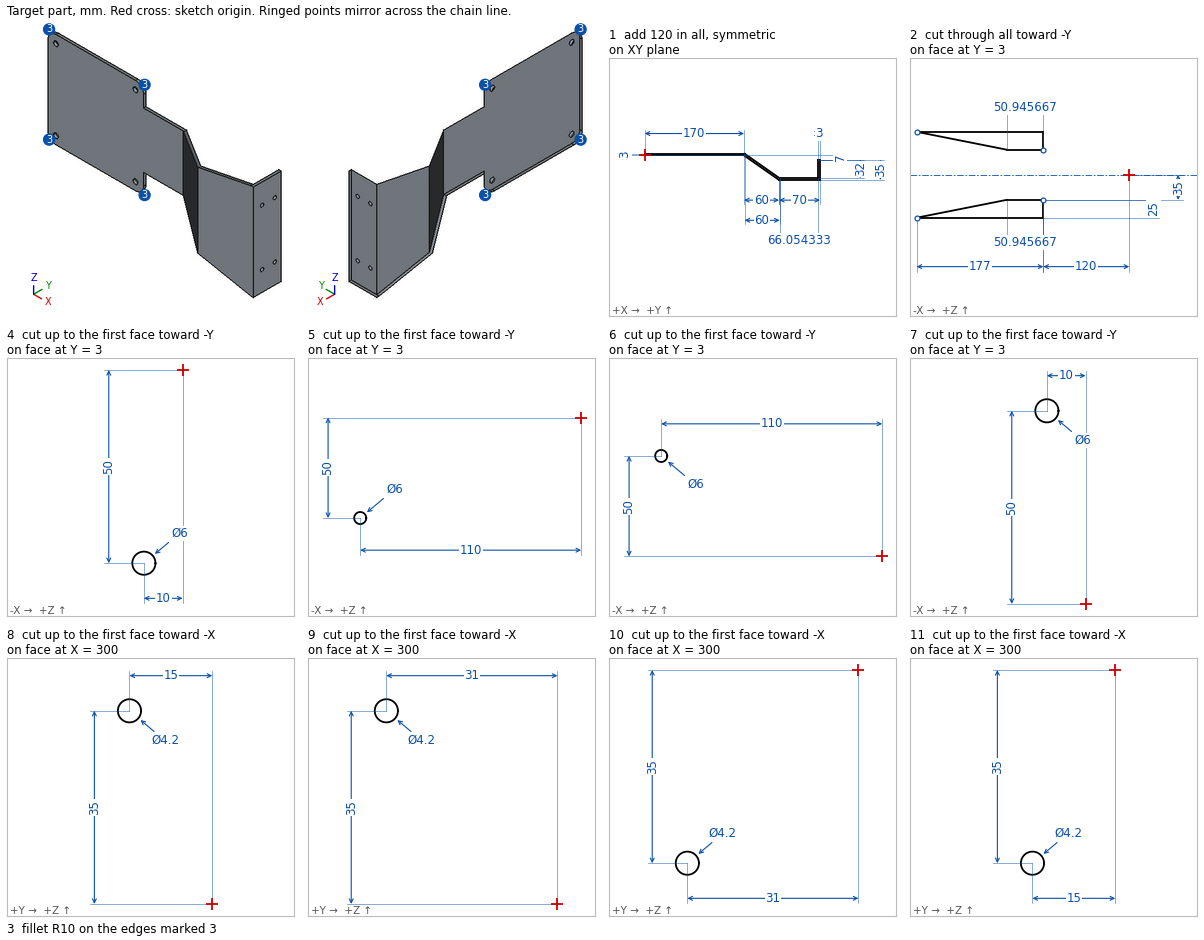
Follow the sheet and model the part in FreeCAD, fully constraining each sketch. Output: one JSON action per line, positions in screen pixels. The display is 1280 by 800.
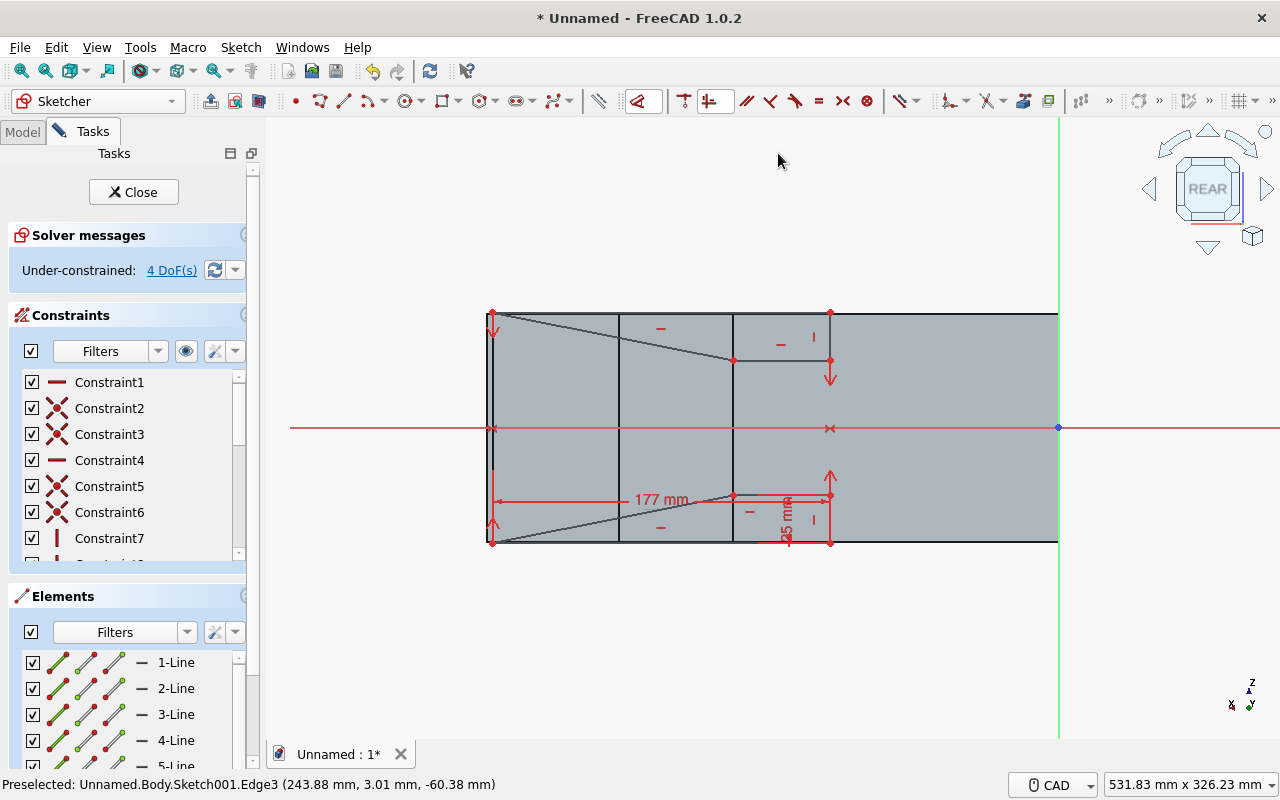
{"action": "left_click", "coordinate": [830, 495]}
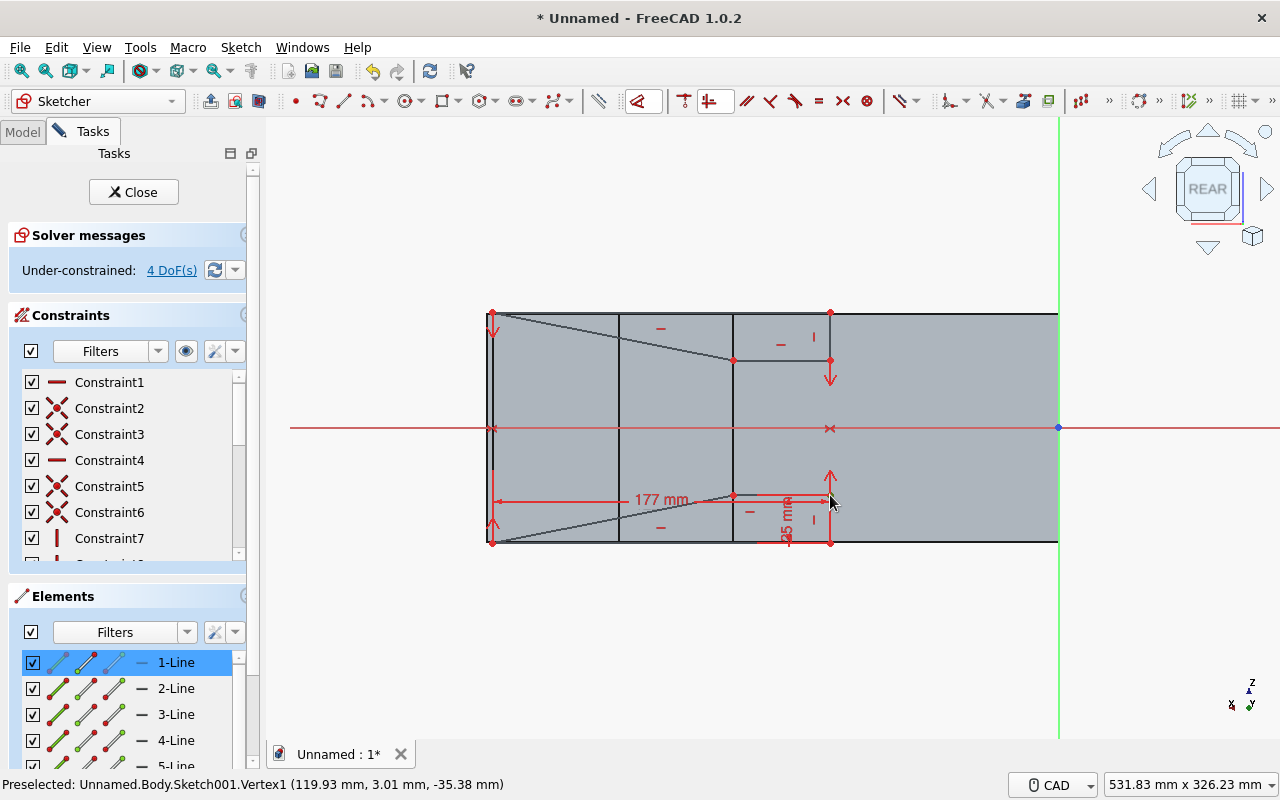
{"action": "key", "text": "i"}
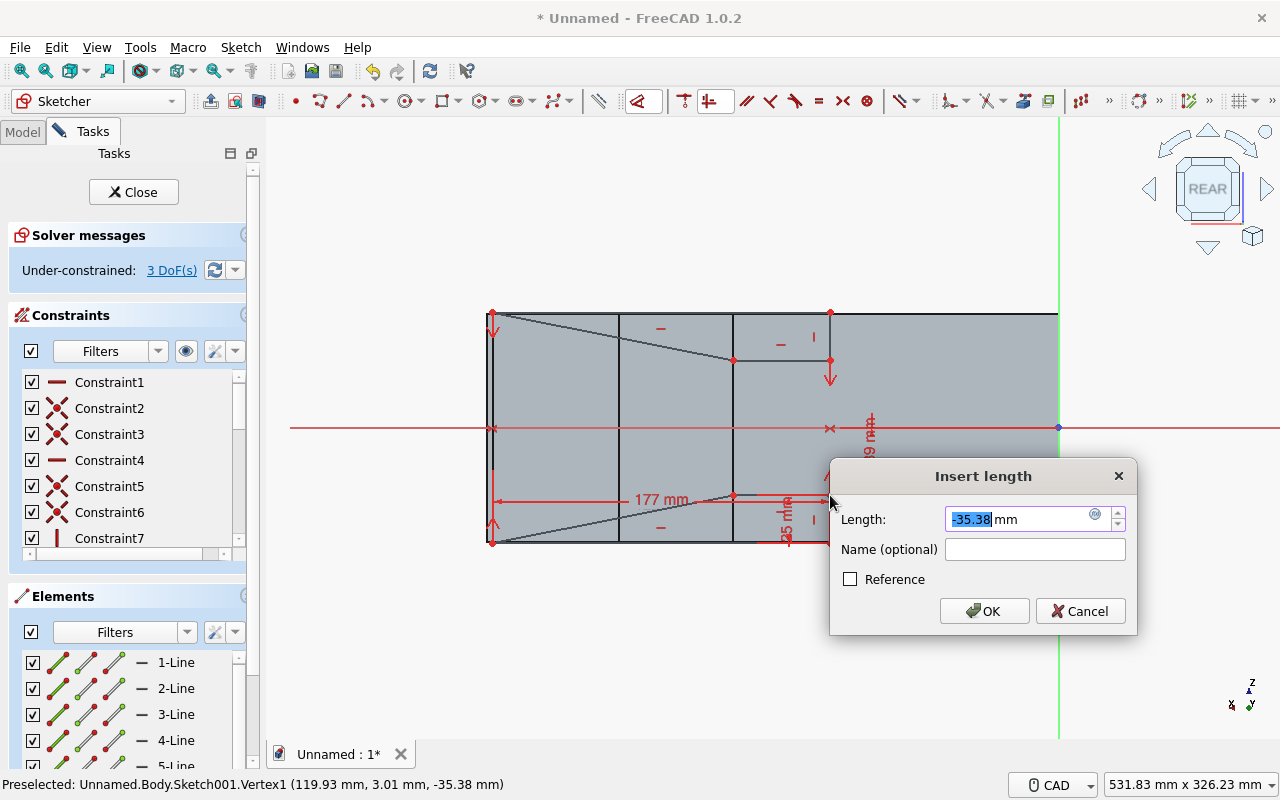
{"action": "type", "text": "-35"}
{"action": "key", "text": "Return"}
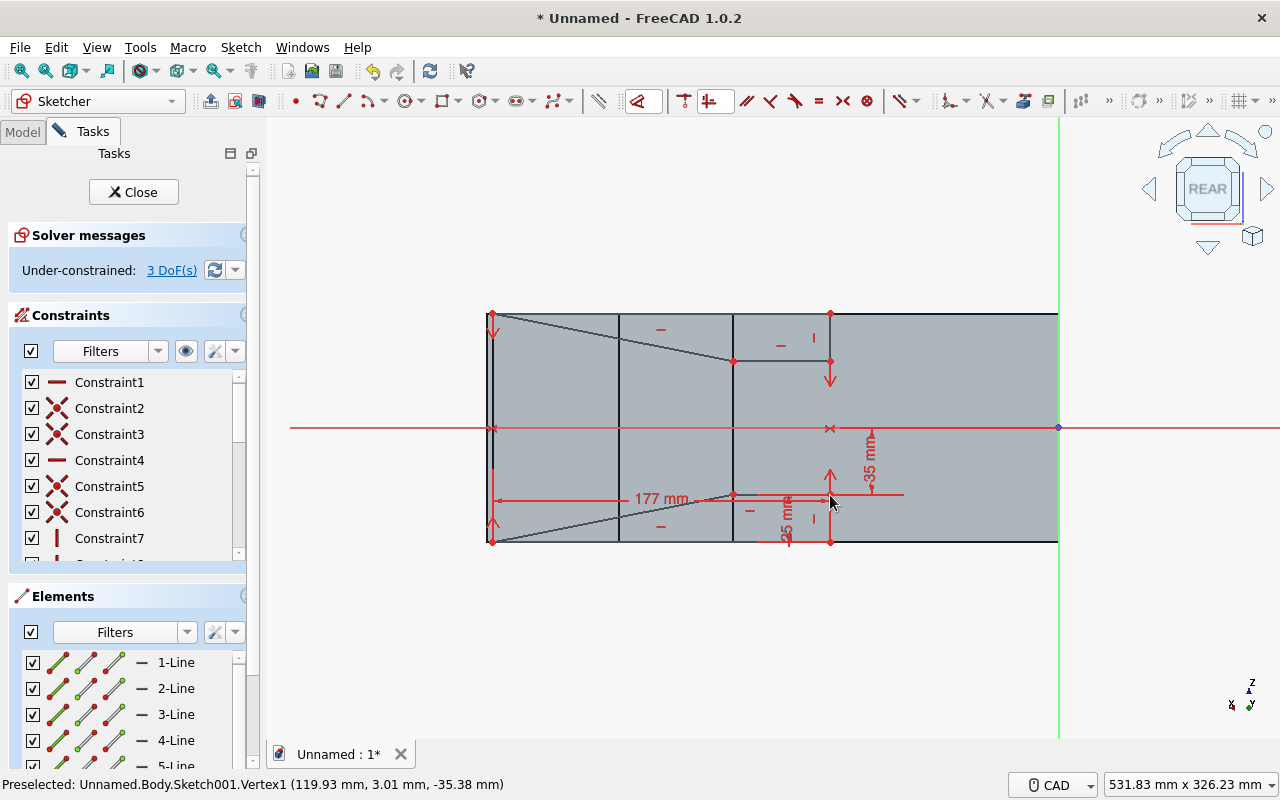
{"action": "left_click", "coordinate": [830, 495]}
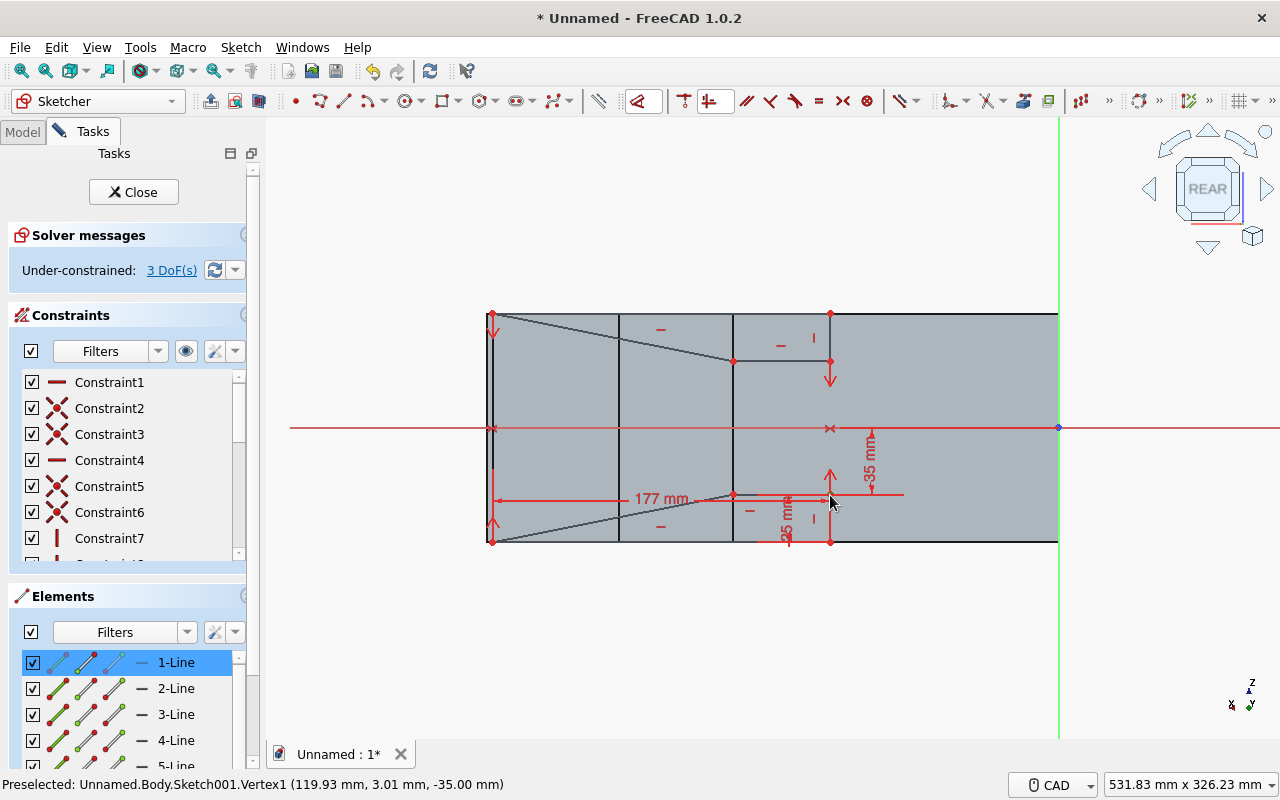
{"action": "left_click", "coordinate": [656, 102]}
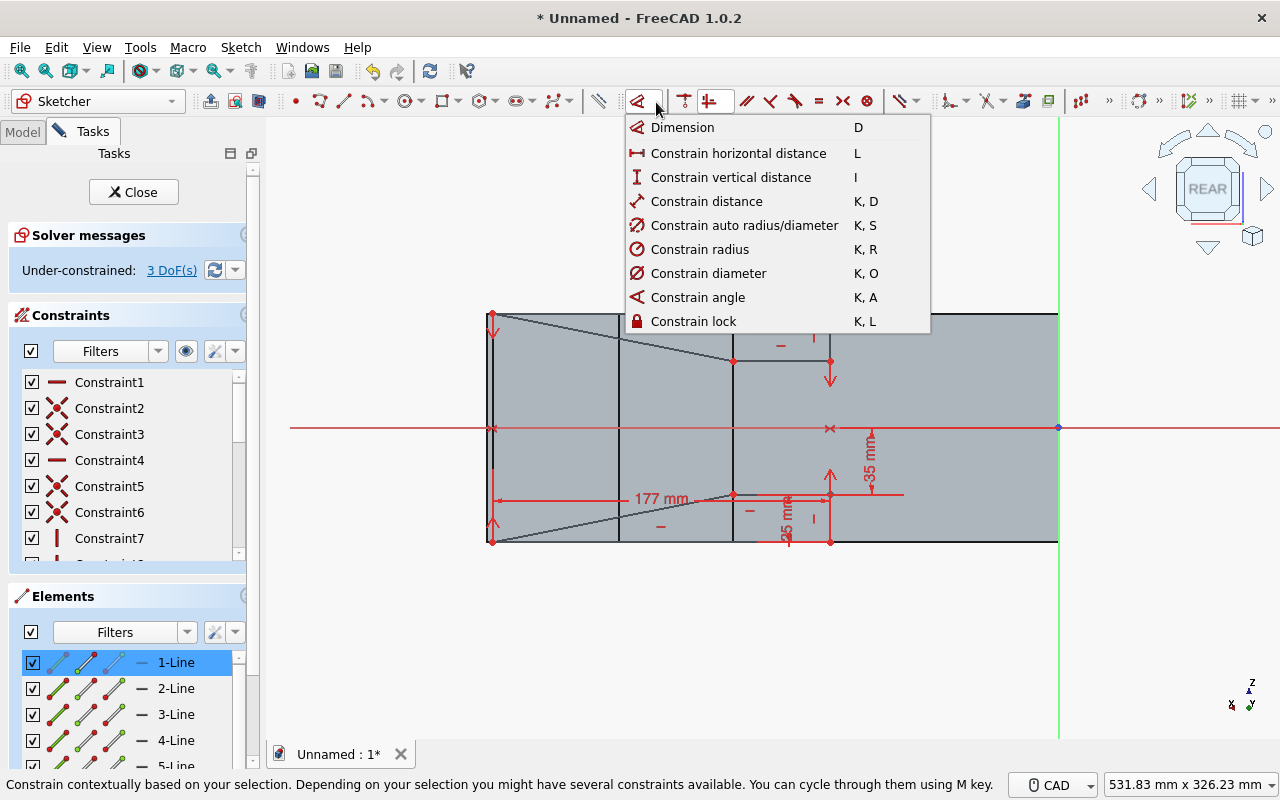
{"action": "left_click", "coordinate": [778, 153]}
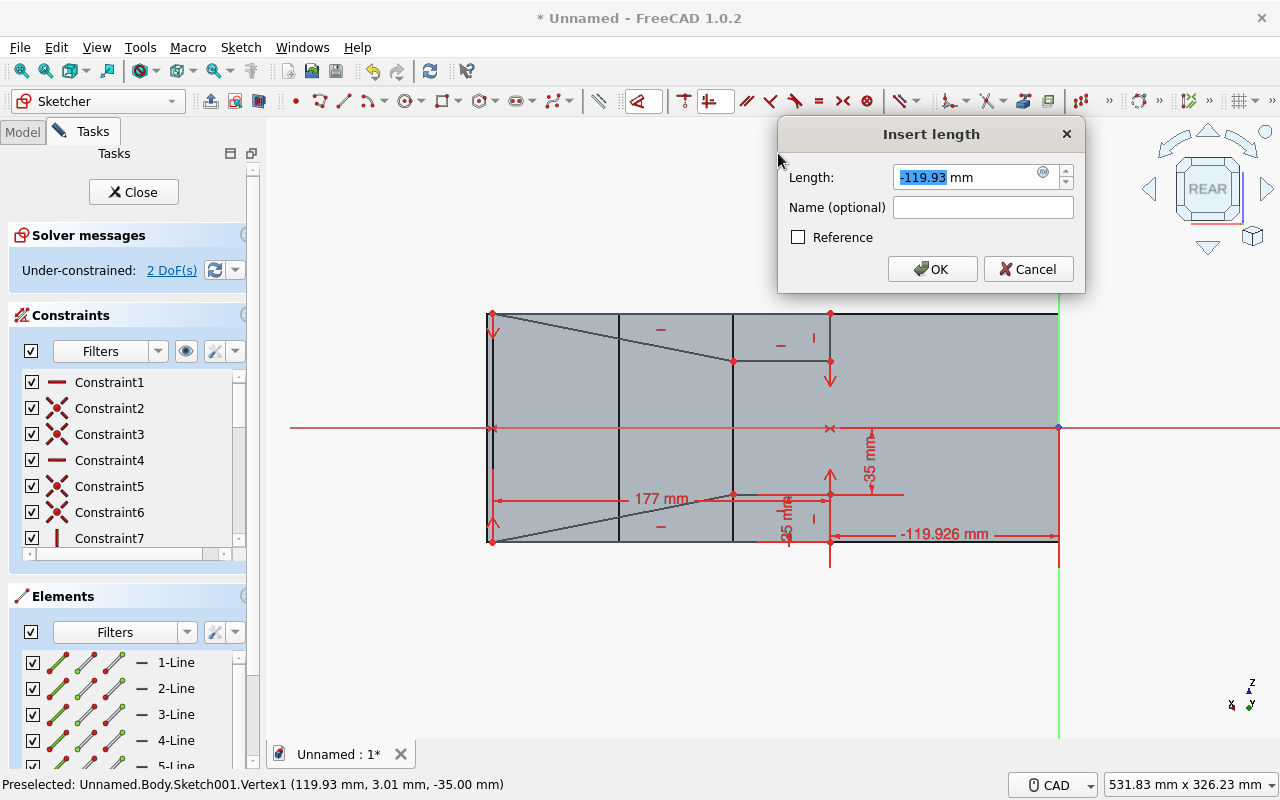
{"action": "type", "text": "-120"}
{"action": "key", "text": "Return"}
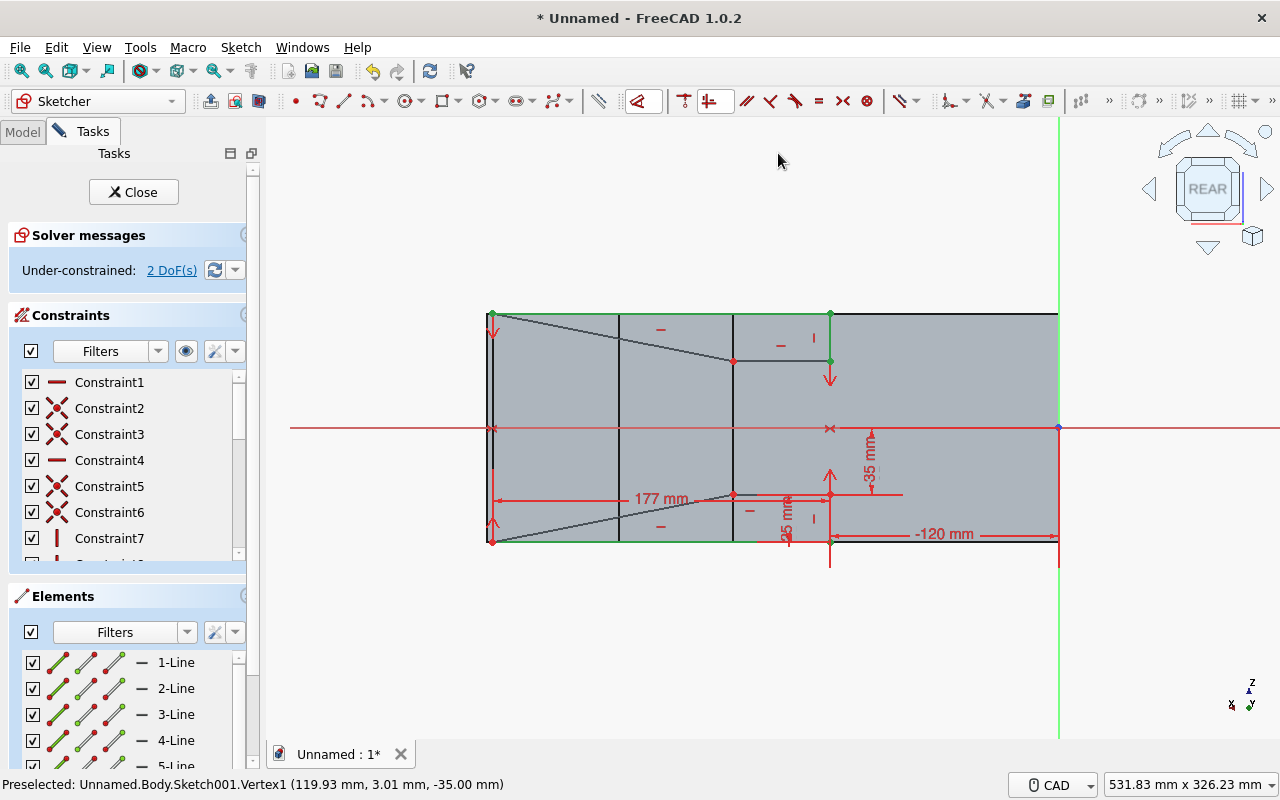
{"action": "left_click", "coordinate": [801, 495]}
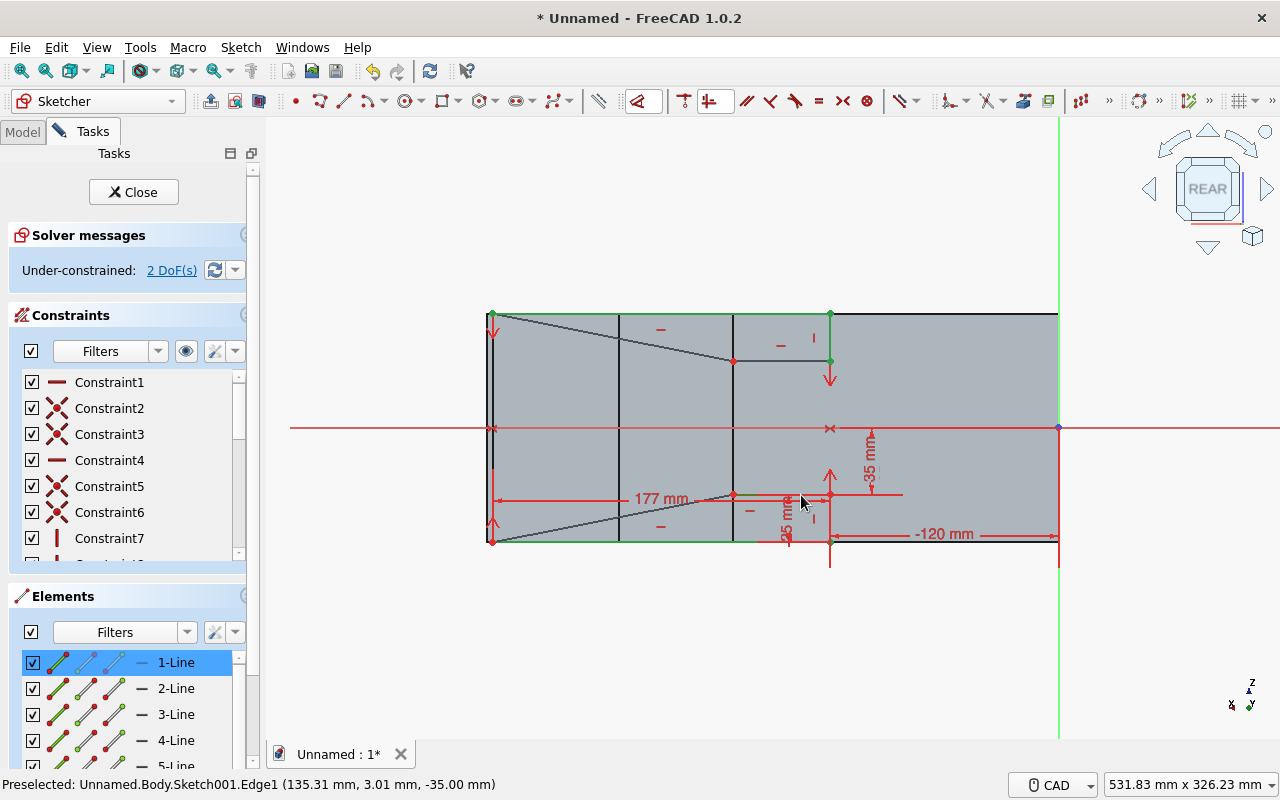
{"action": "key", "text": "l"}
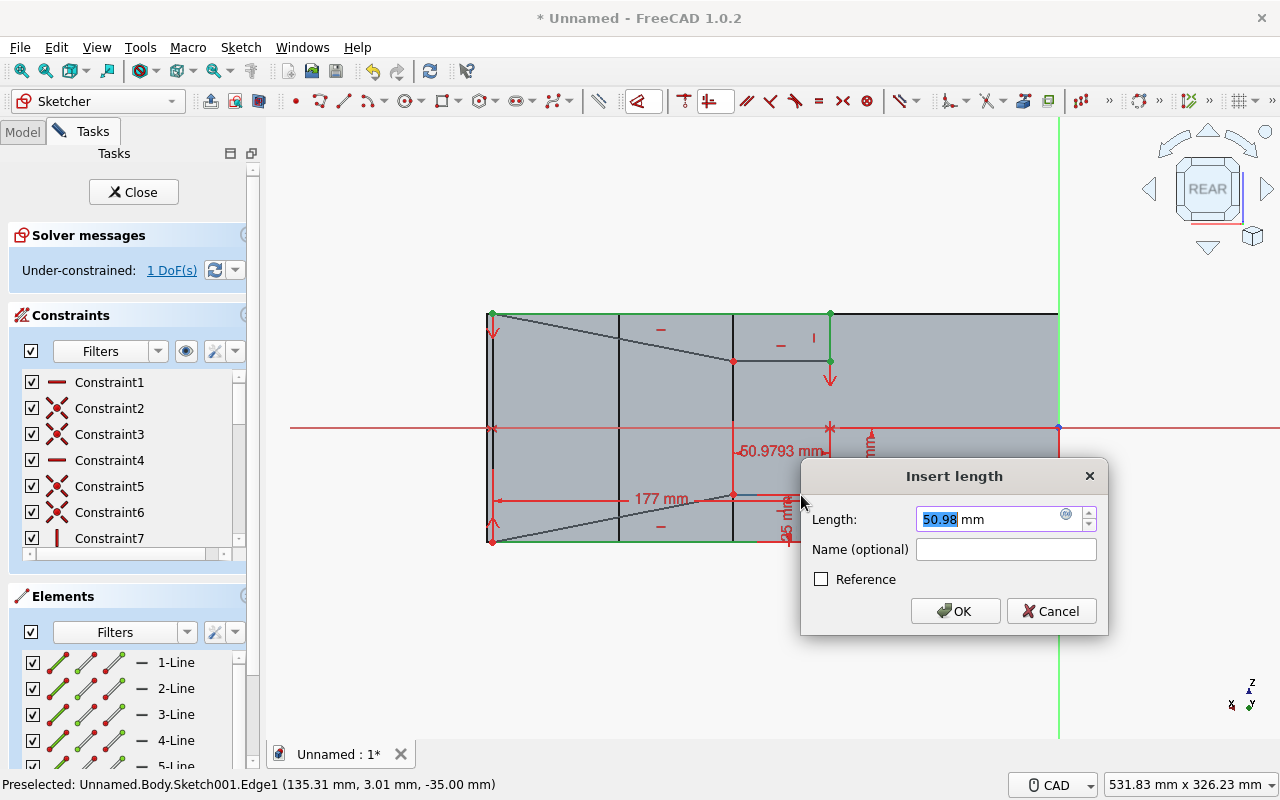
{"action": "type", "text": "50.945667"}
{"action": "key", "text": "Return"}